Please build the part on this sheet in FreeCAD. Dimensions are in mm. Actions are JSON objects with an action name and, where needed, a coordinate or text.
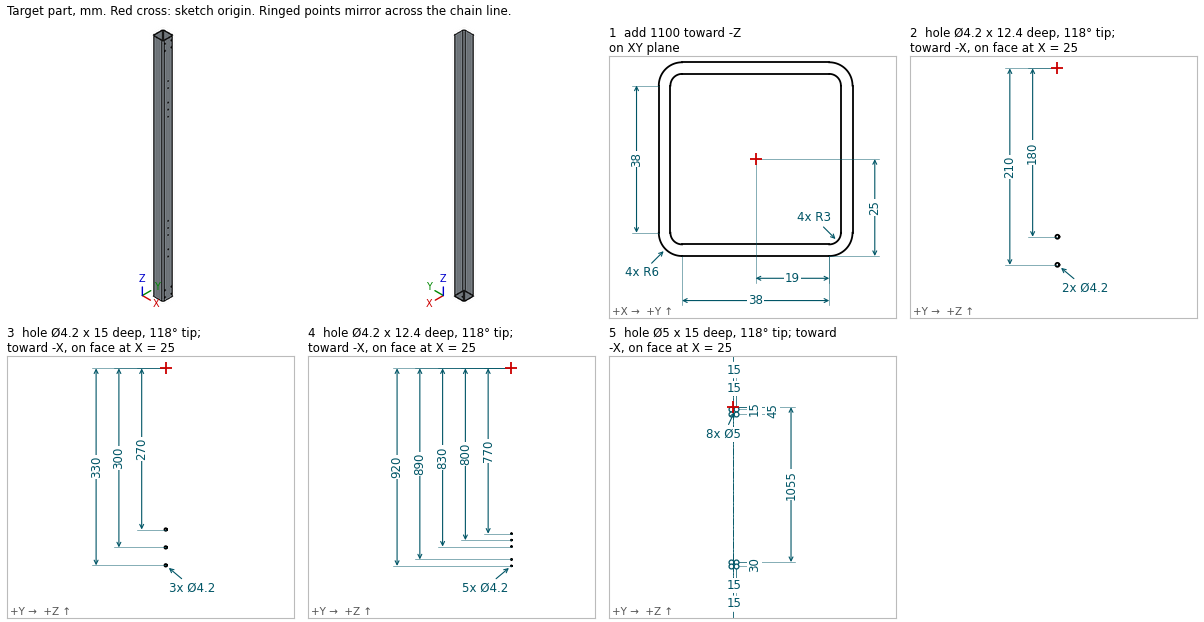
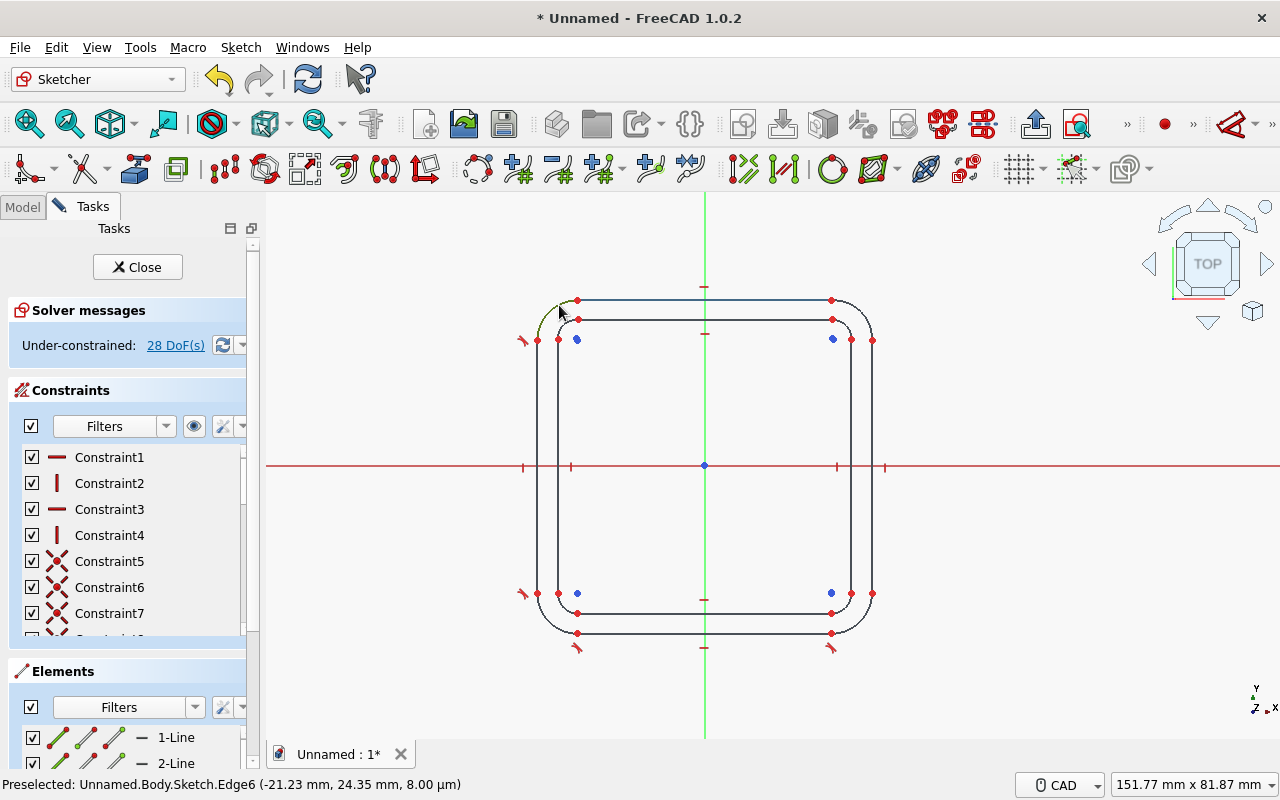
{"action": "key", "text": "t"}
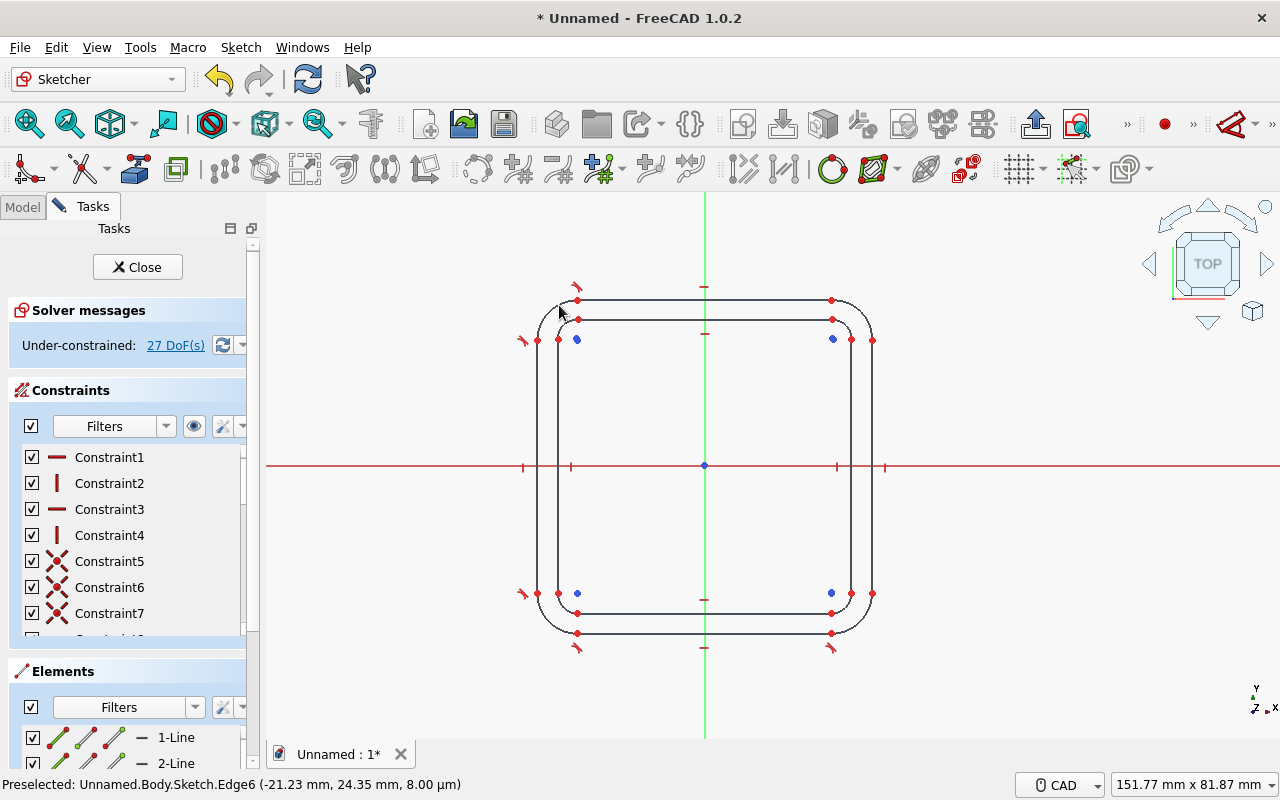
{"action": "left_click", "coordinate": [654, 300]}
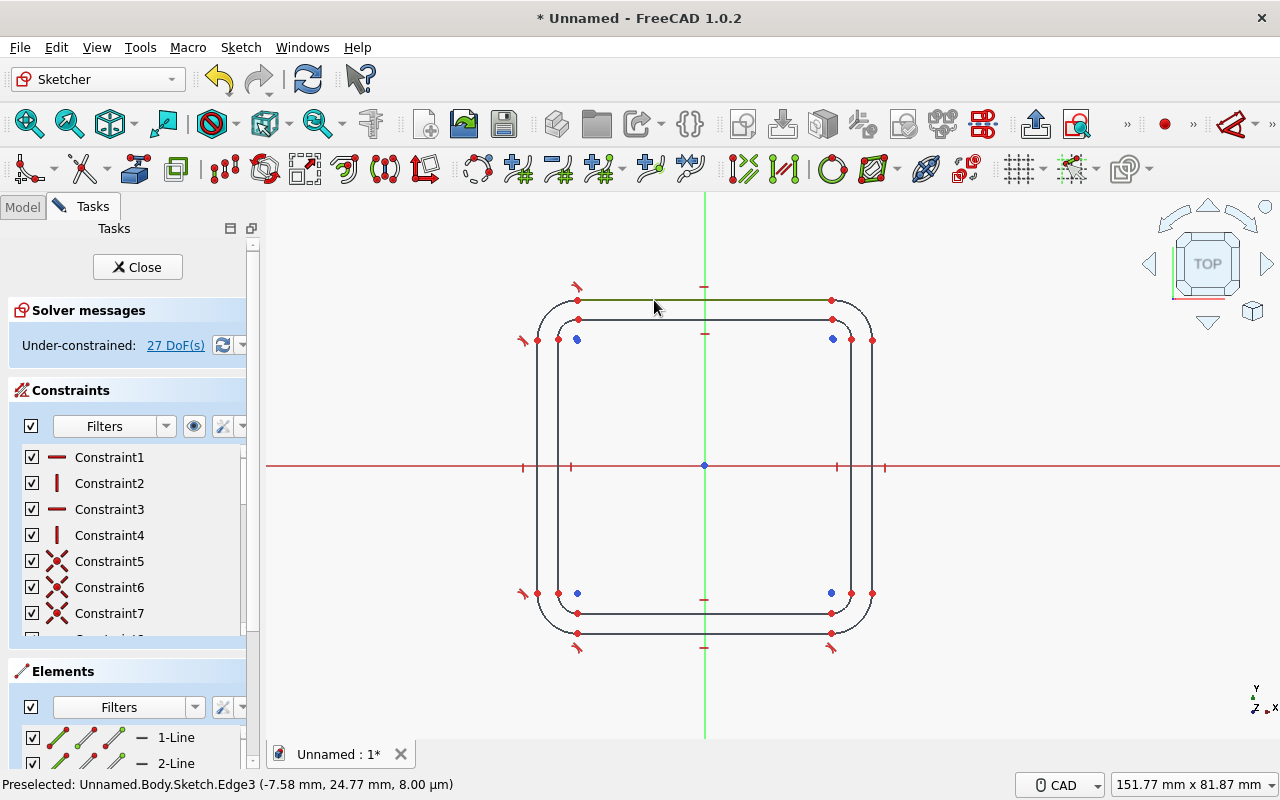
{"action": "left_click", "coordinate": [868, 322]}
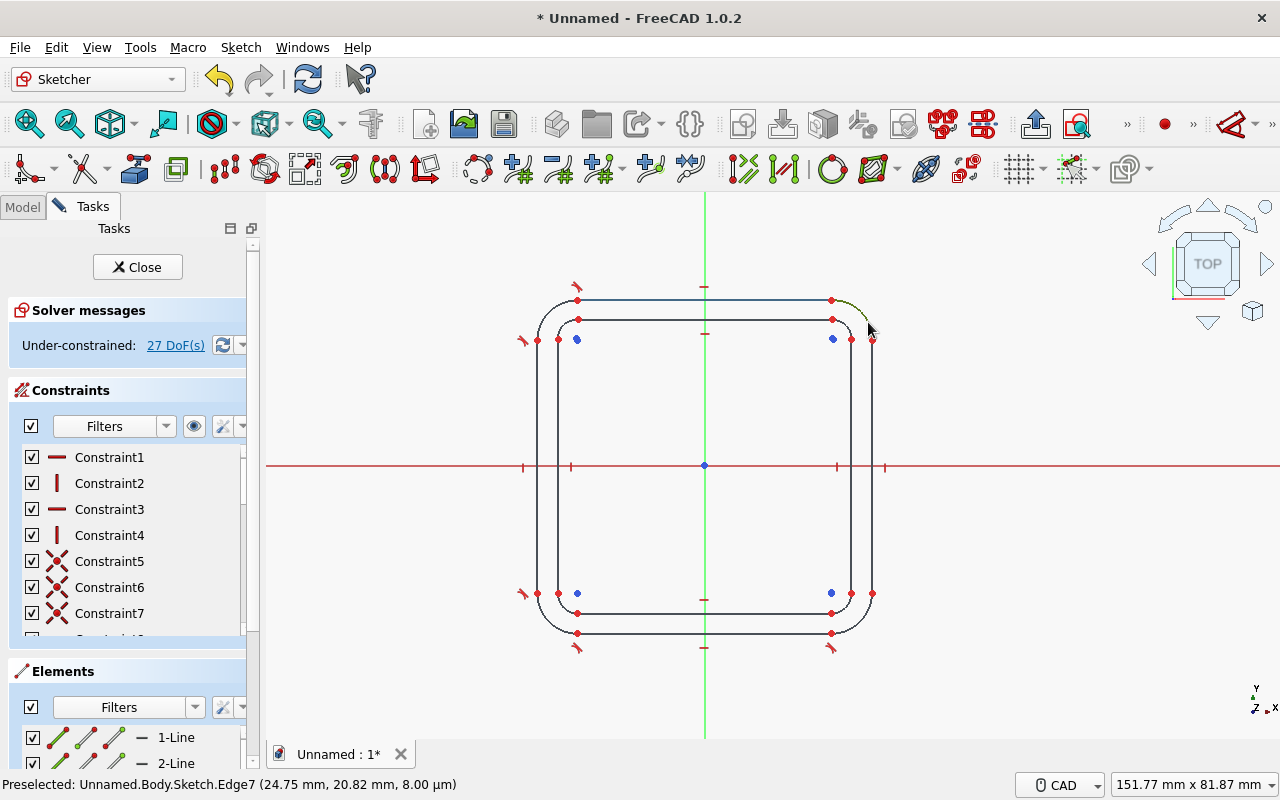
{"action": "key", "text": "t"}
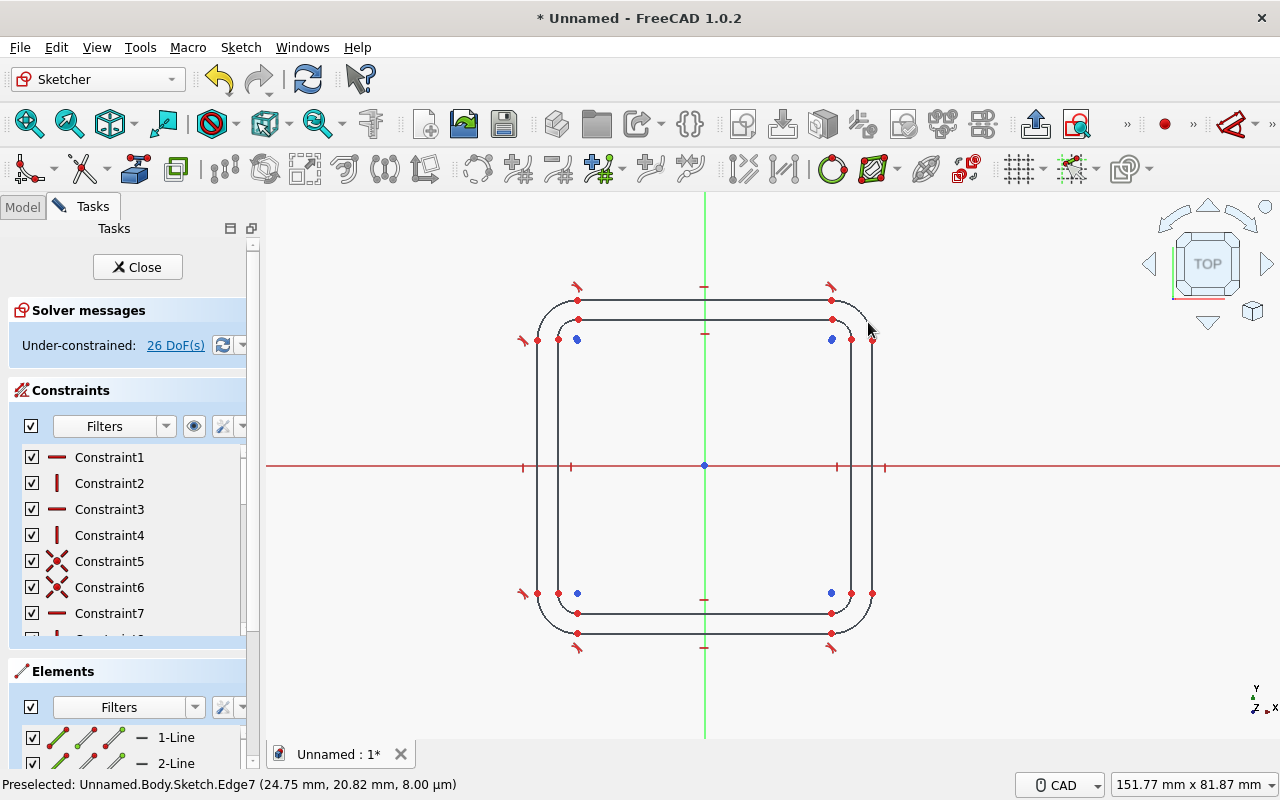
{"action": "left_click", "coordinate": [872, 416]}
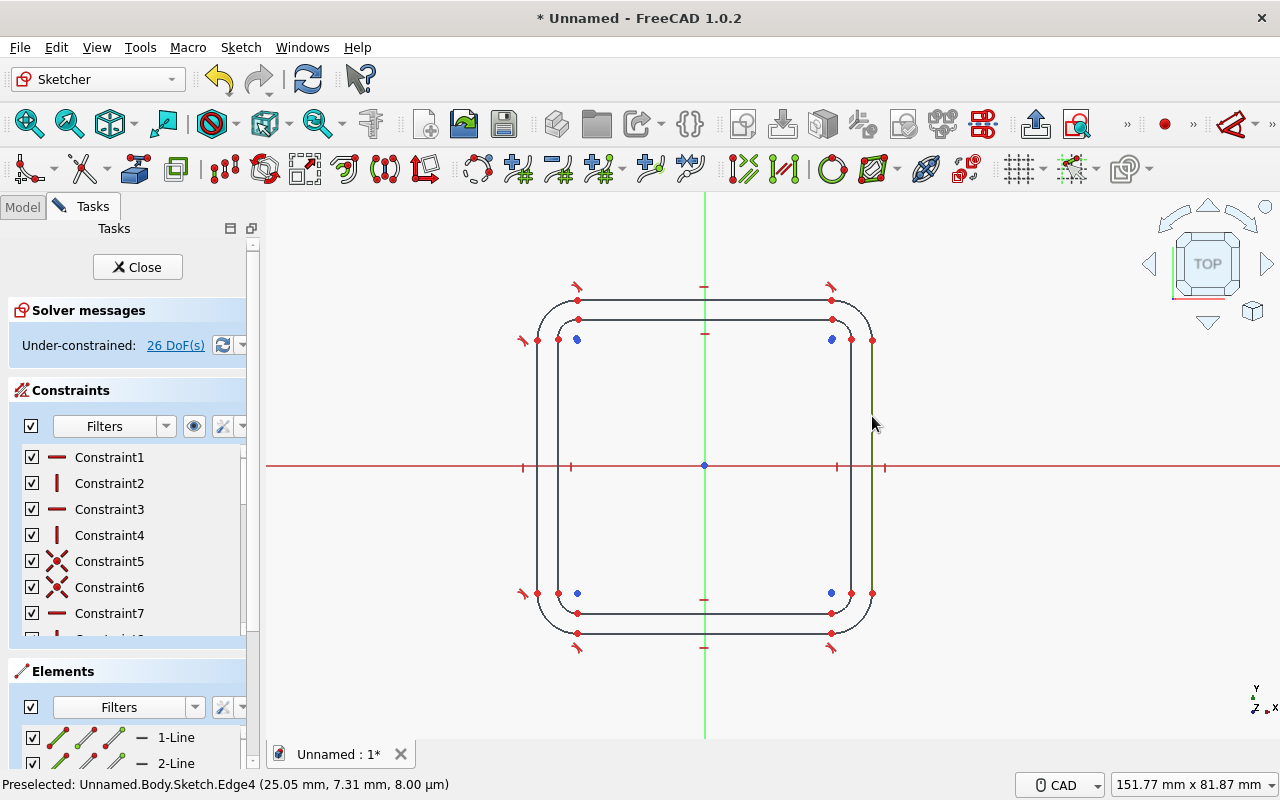
{"action": "left_click", "coordinate": [868, 322]}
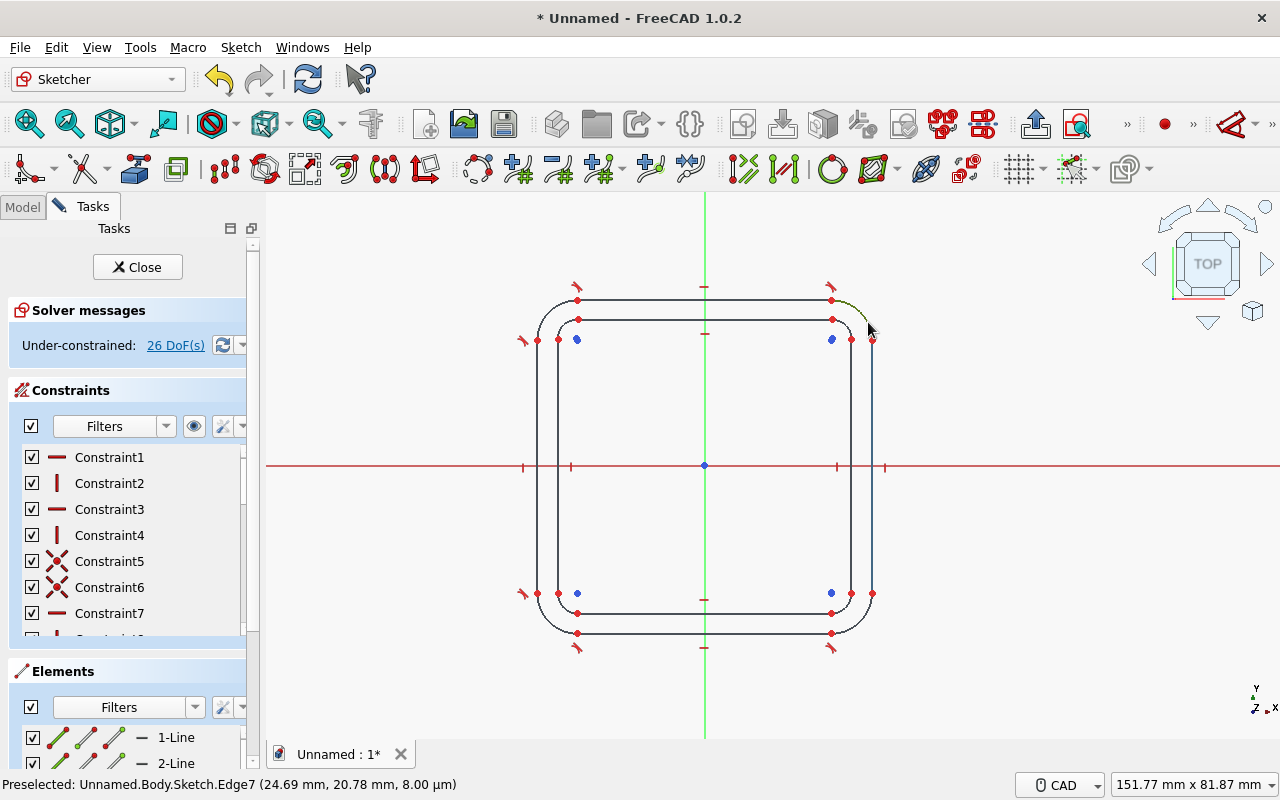
{"action": "key", "text": "t"}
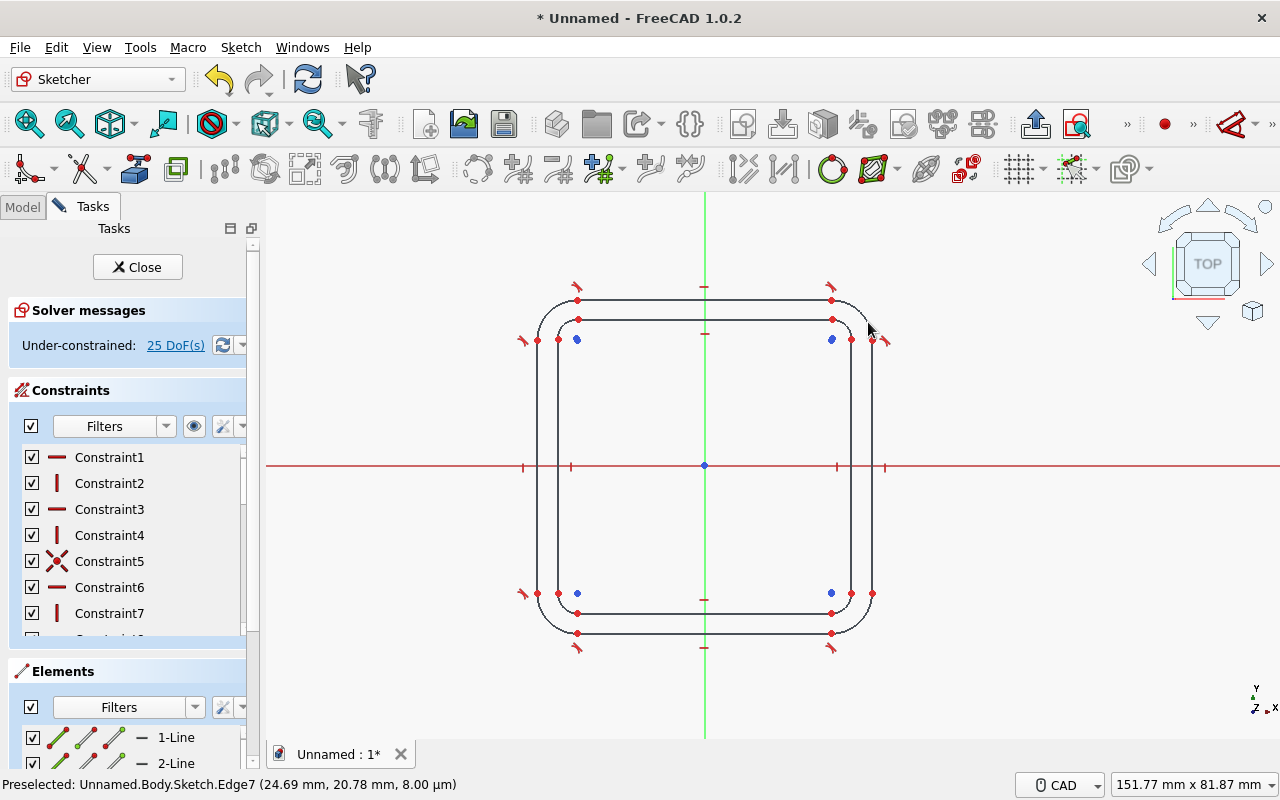
{"action": "left_click", "coordinate": [872, 416]}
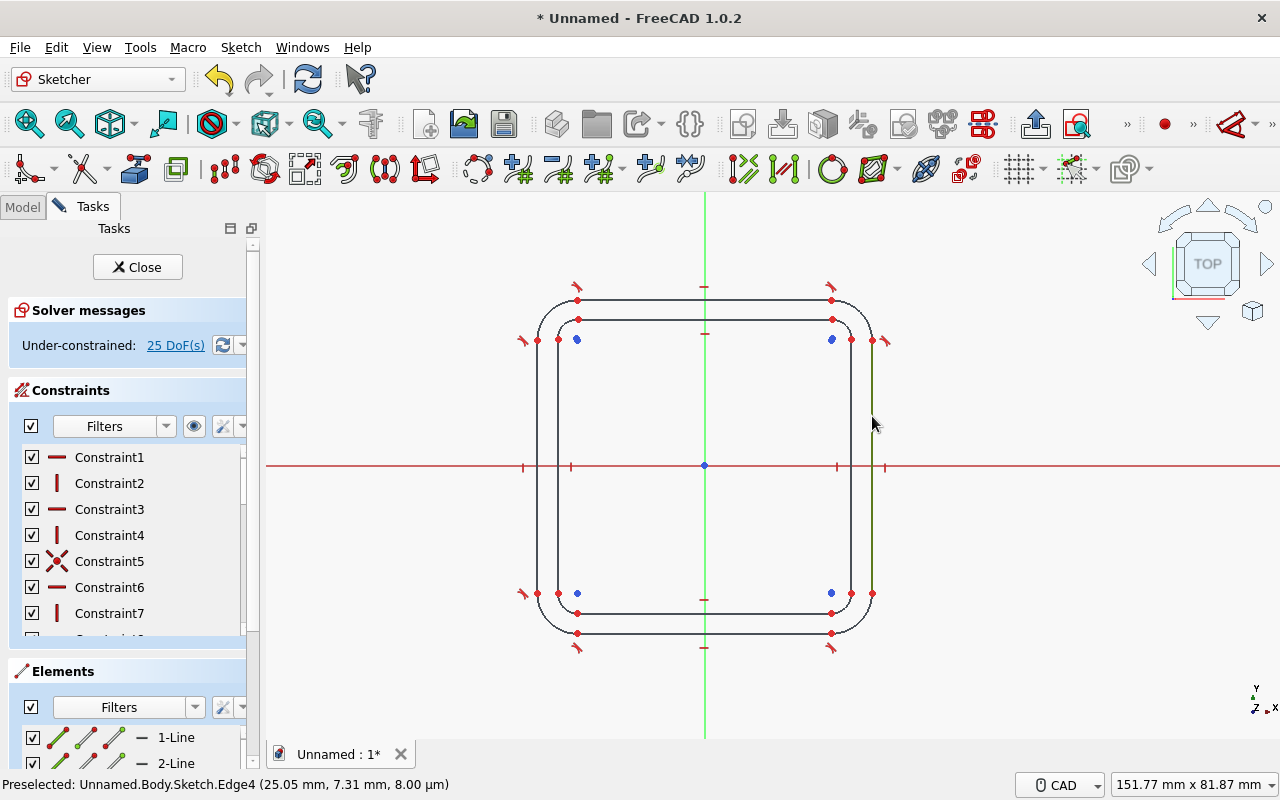
{"action": "left_click", "coordinate": [849, 629]}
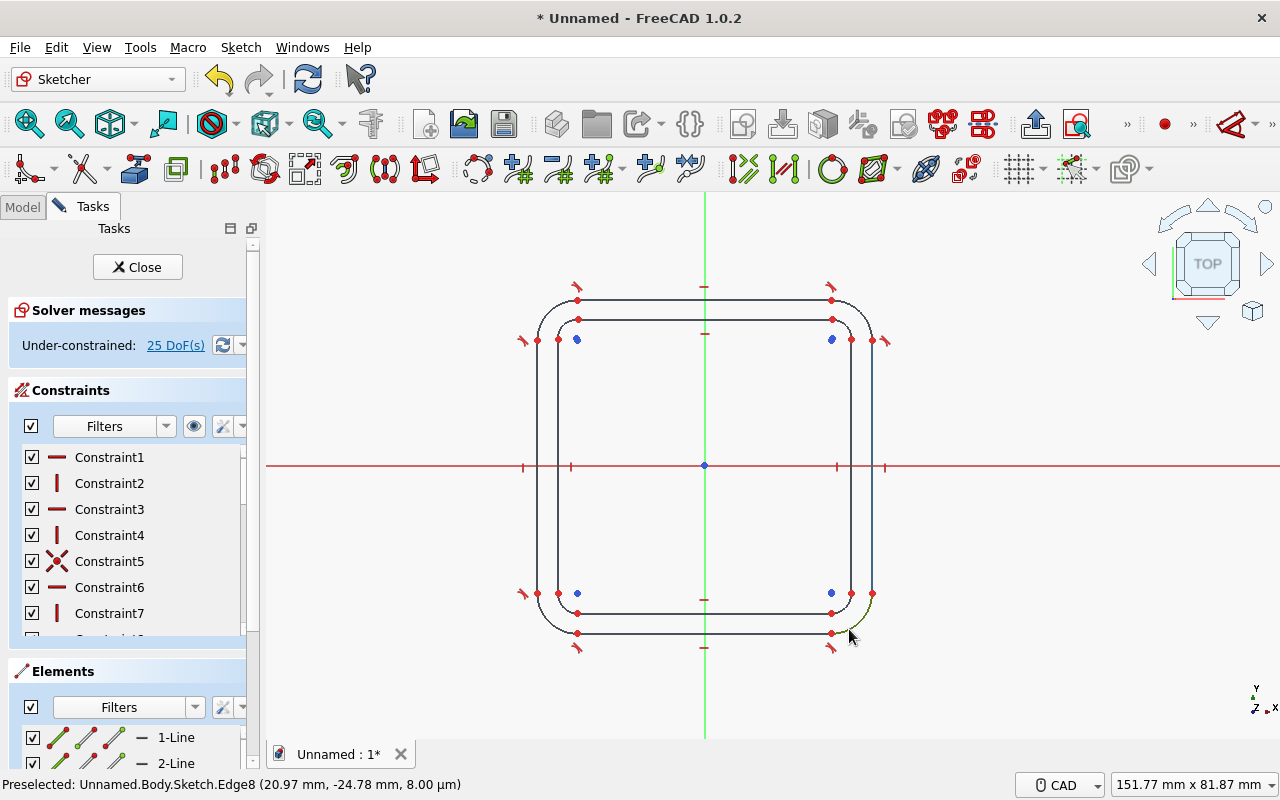
{"action": "key", "text": "t"}